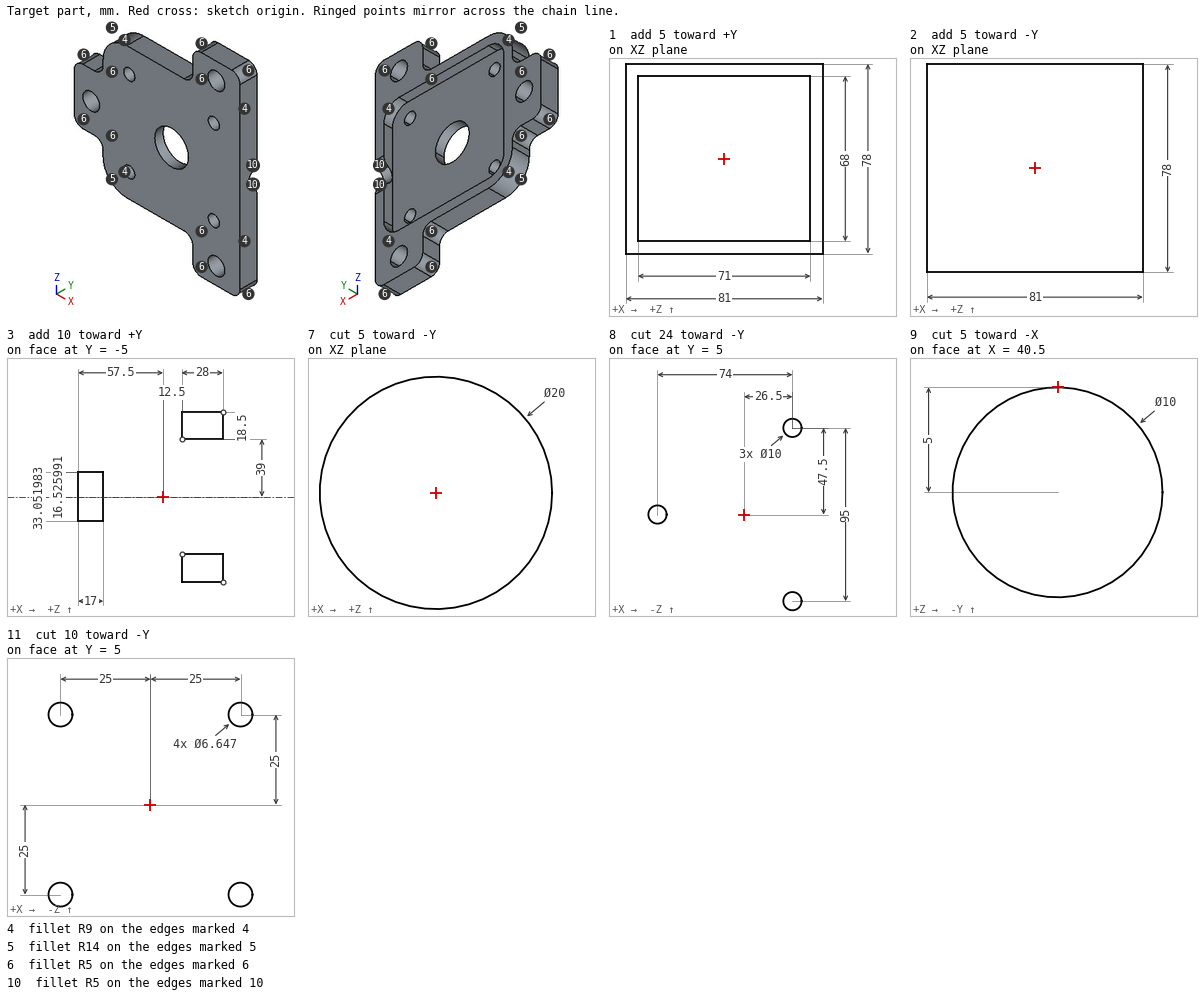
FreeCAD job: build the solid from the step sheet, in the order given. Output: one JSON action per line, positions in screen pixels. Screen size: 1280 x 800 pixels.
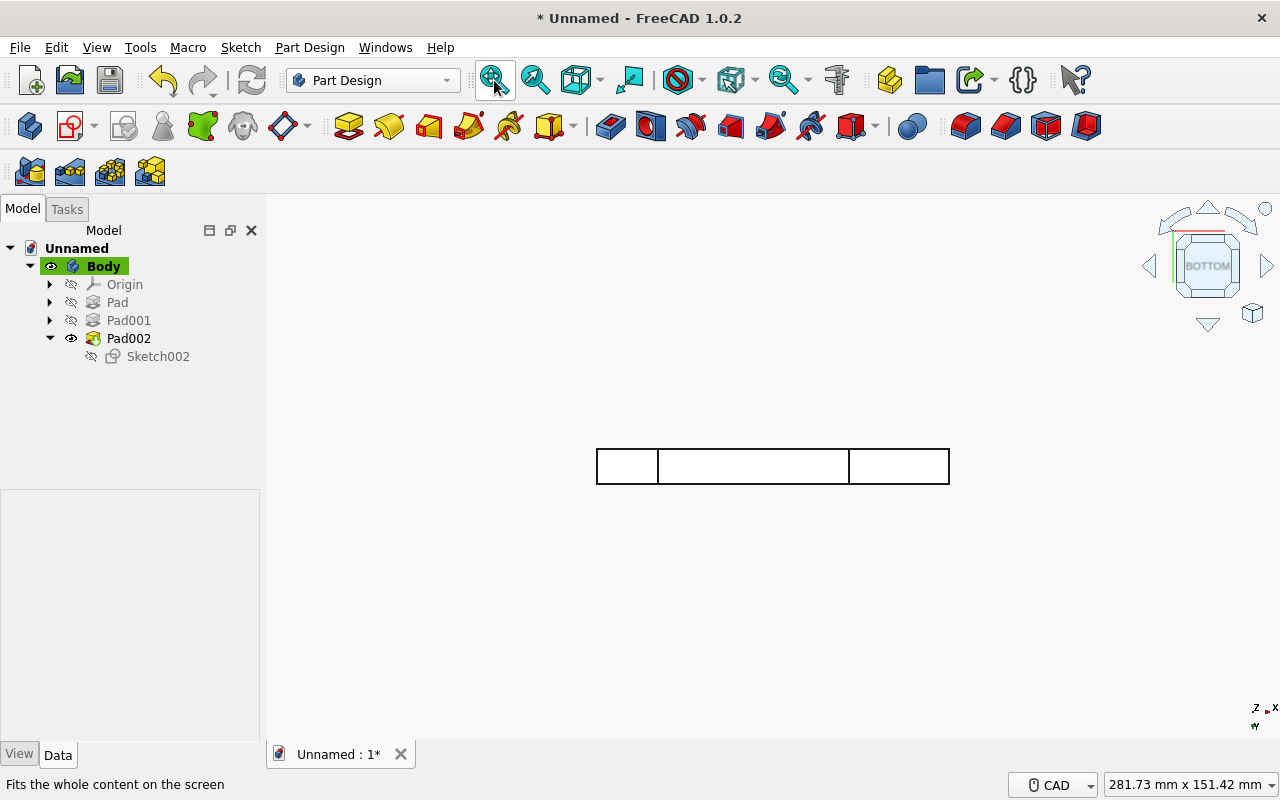
{"action": "scroll", "coordinate": [931, 474], "scroll_direction": "up", "scroll_amount": 4}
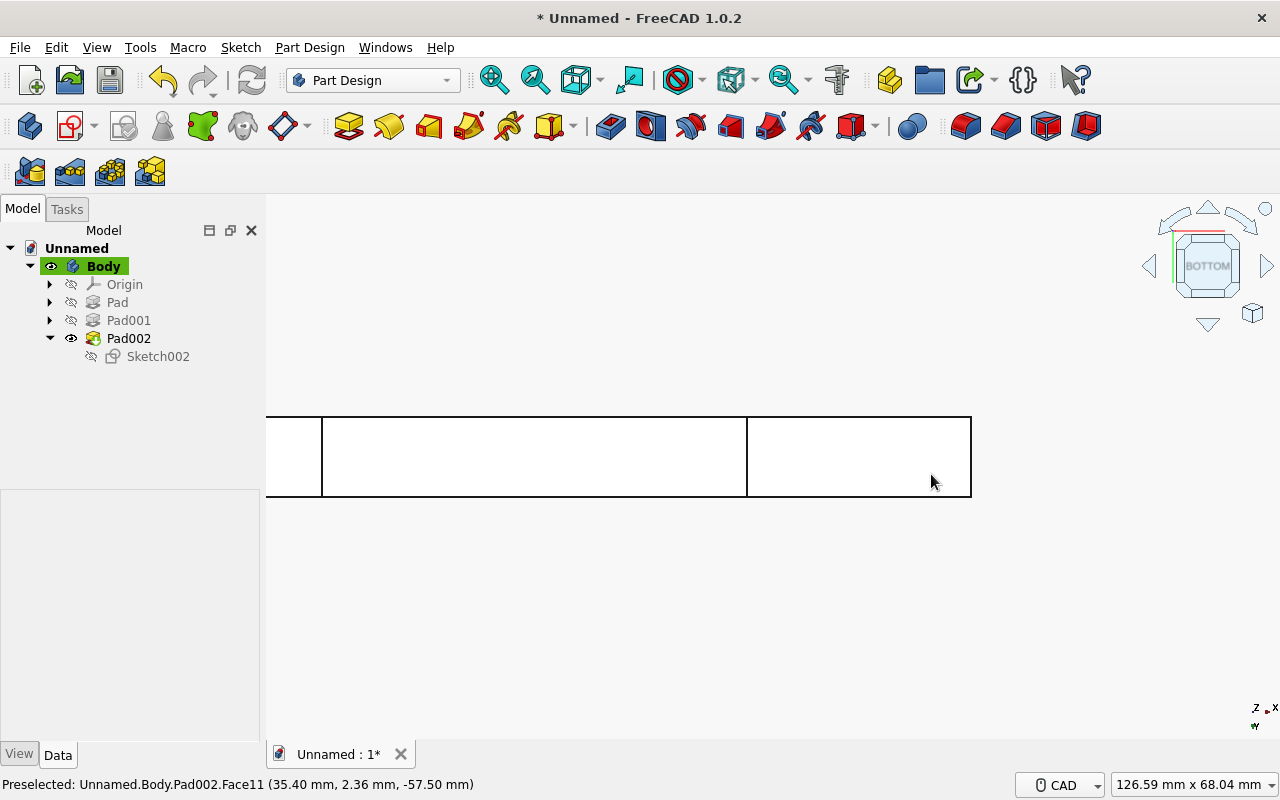
{"action": "key", "text": "v f"}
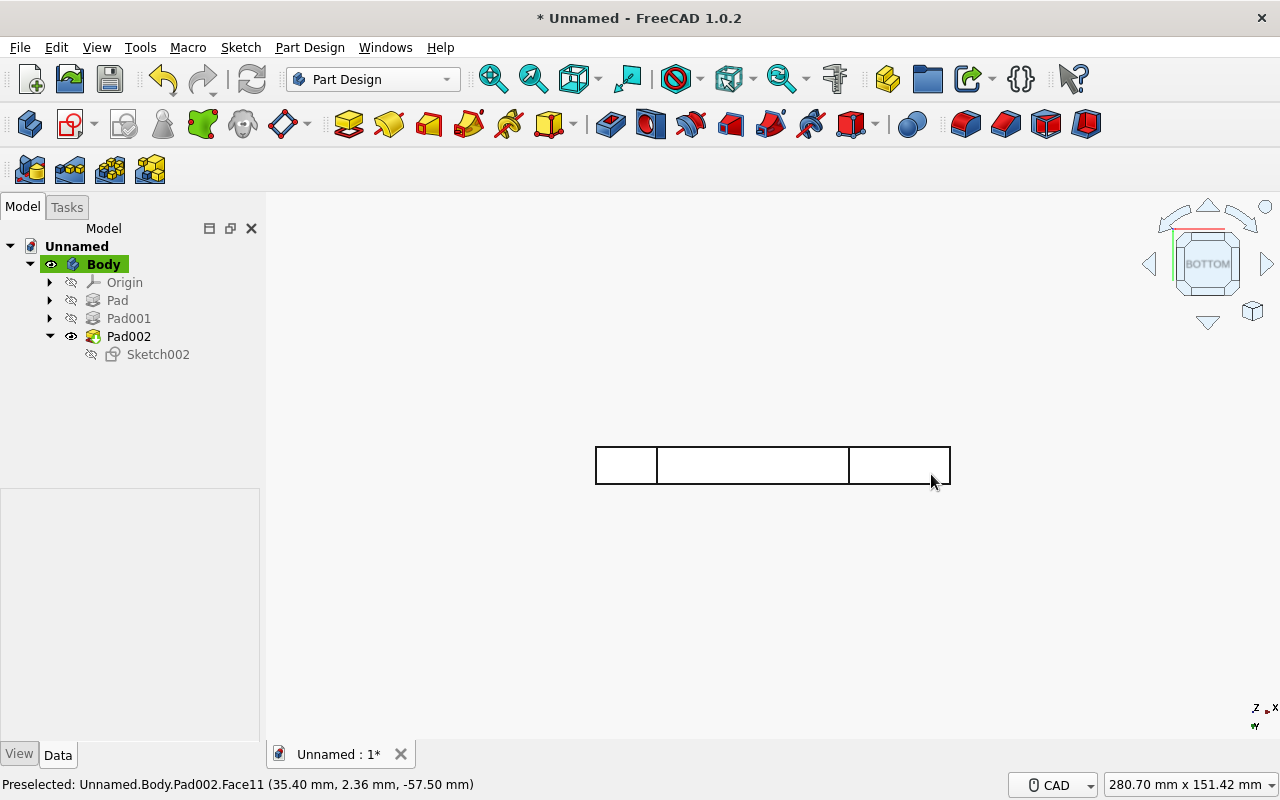
{"action": "key", "text": "4"}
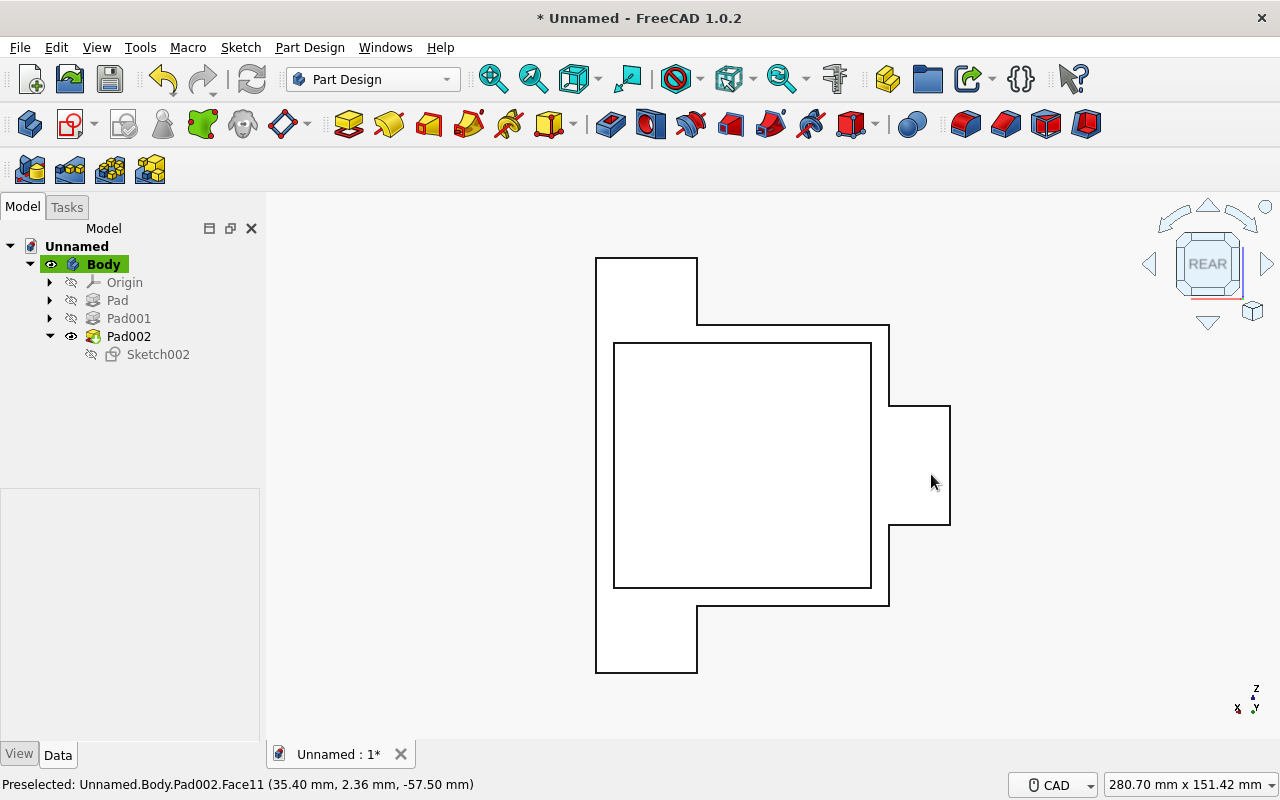
{"action": "scroll", "coordinate": [614, 342], "scroll_direction": "up", "scroll_amount": 4}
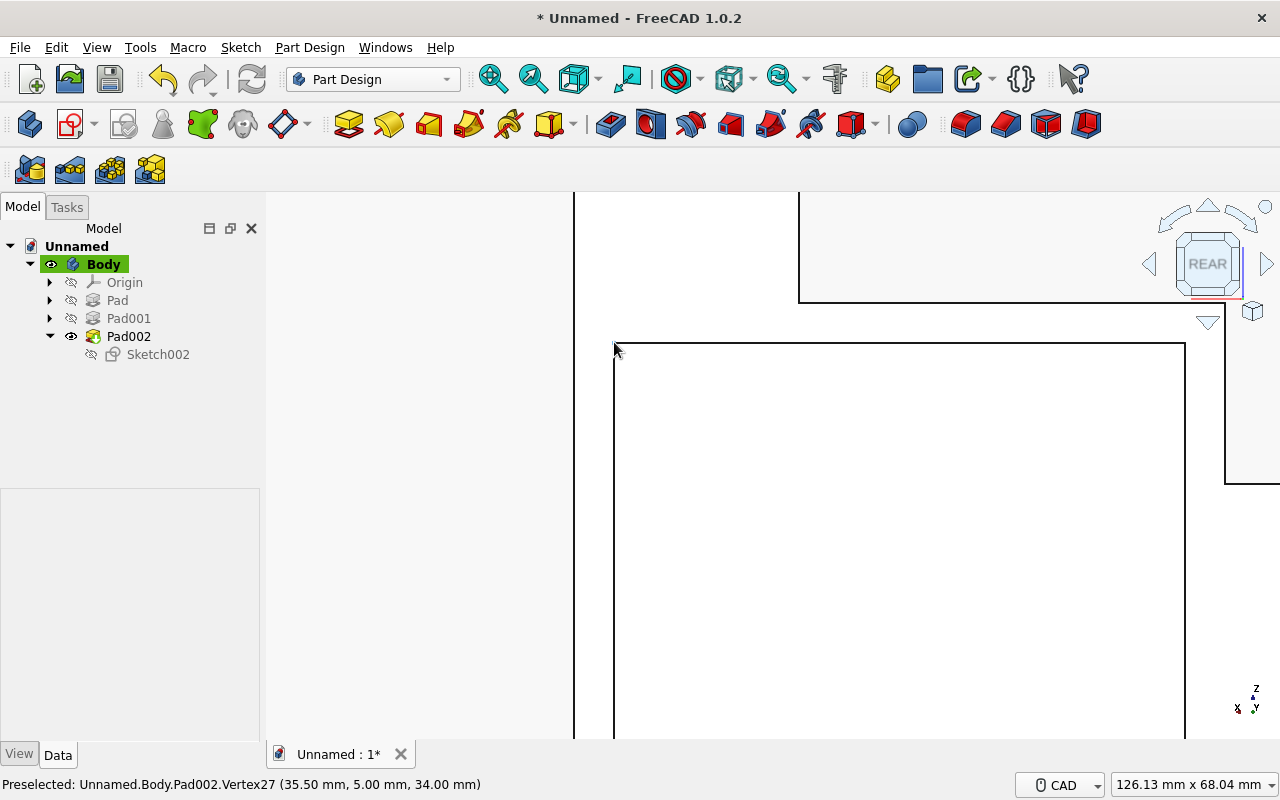
{"action": "key", "text": "v f"}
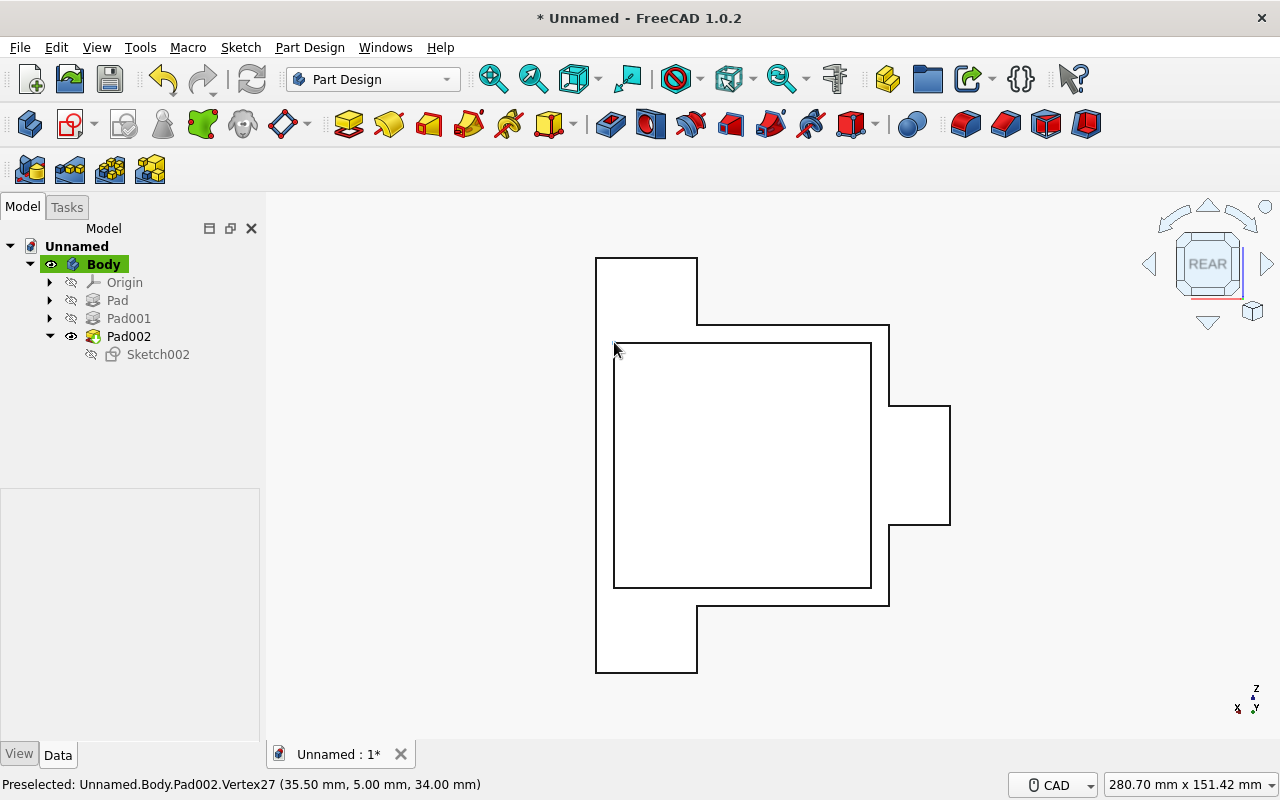
{"action": "key", "text": "6"}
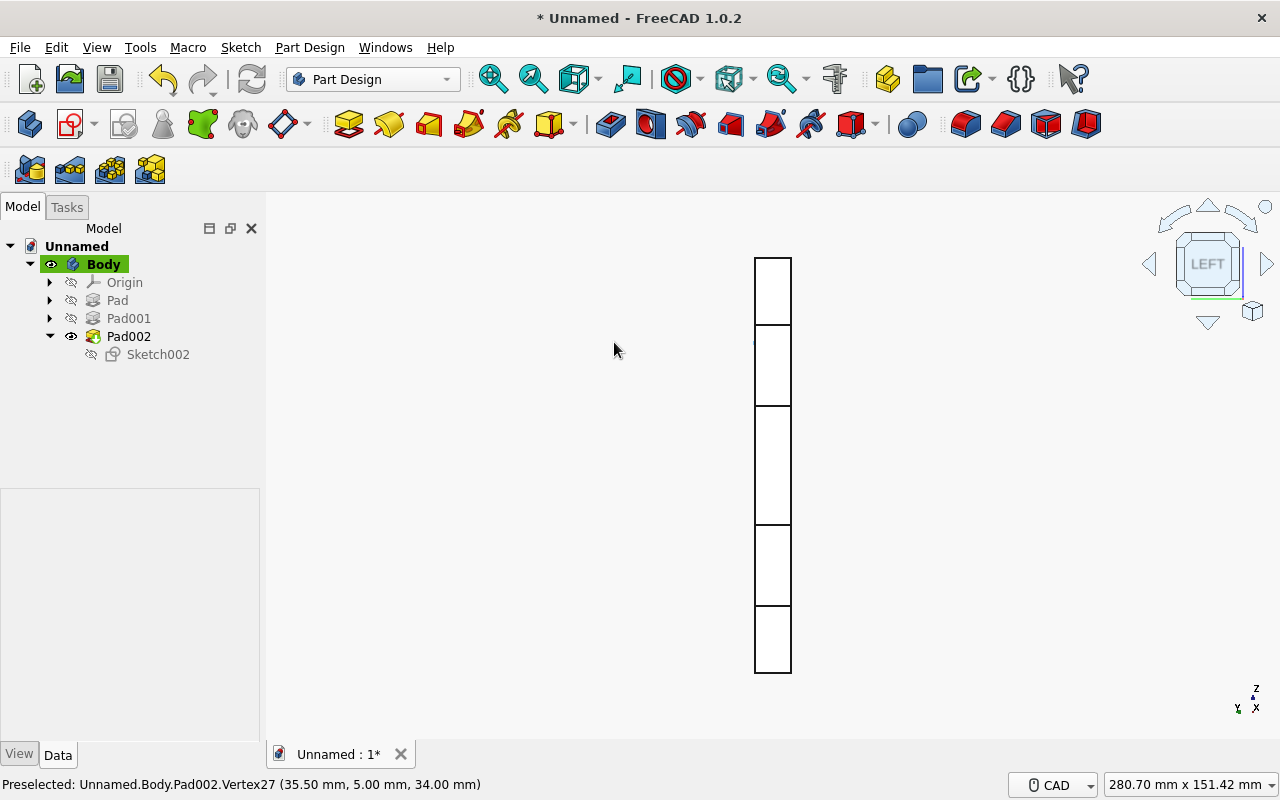
{"action": "scroll", "coordinate": [764, 342], "scroll_direction": "up", "scroll_amount": 4}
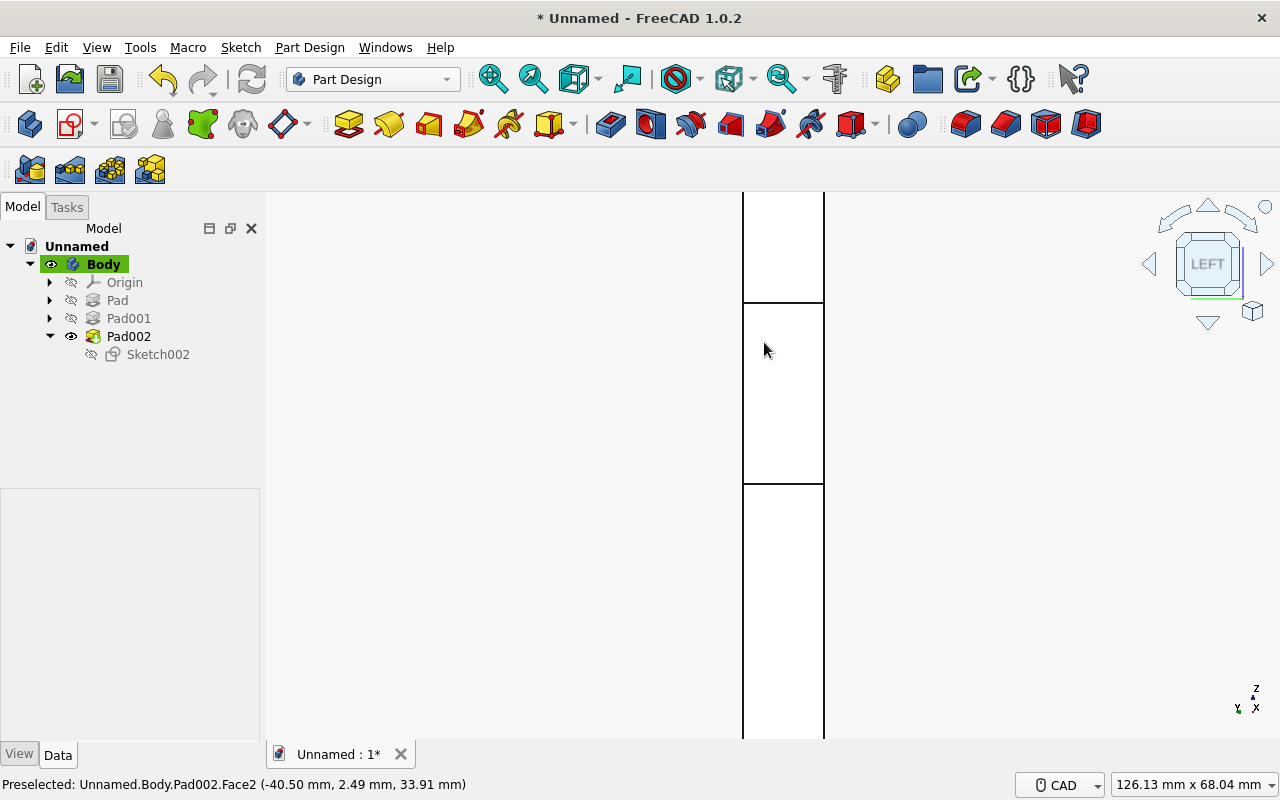
{"action": "left_click", "coordinate": [494, 80]}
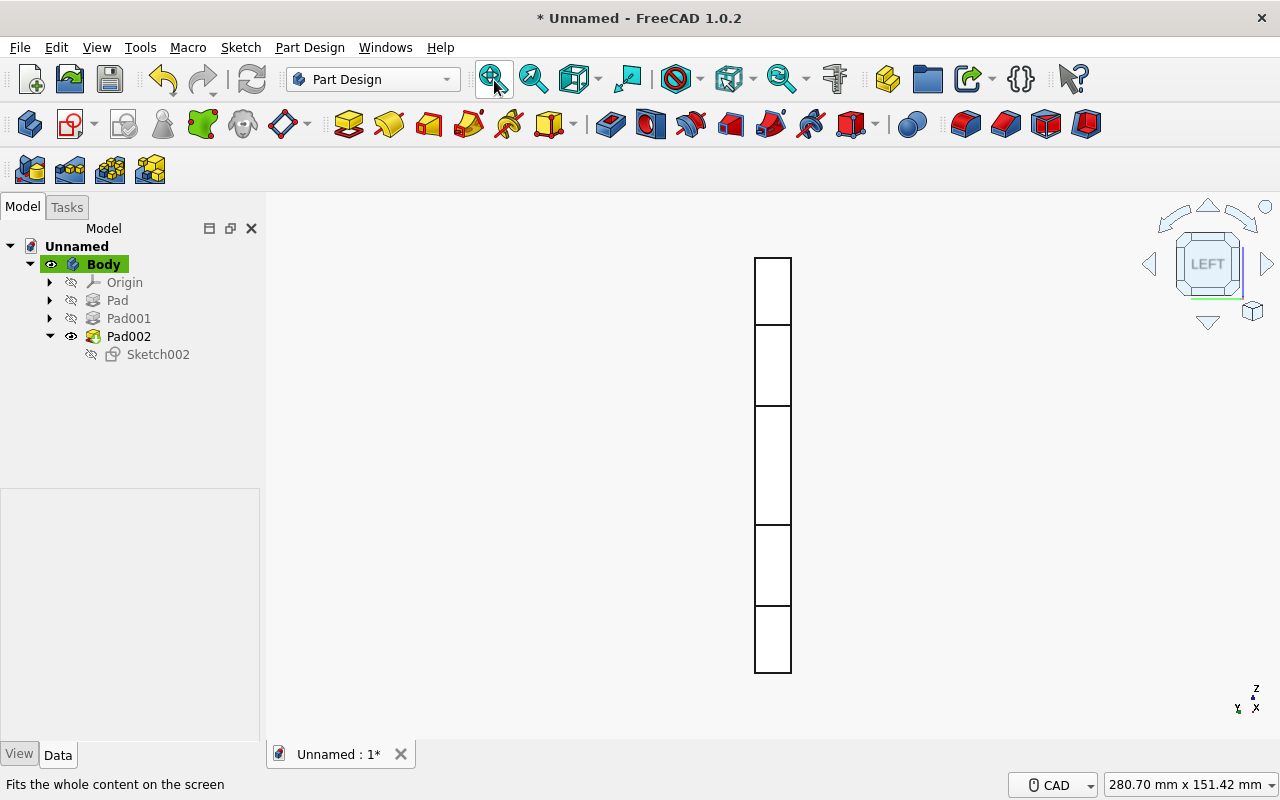
{"action": "key", "text": "v 3"}